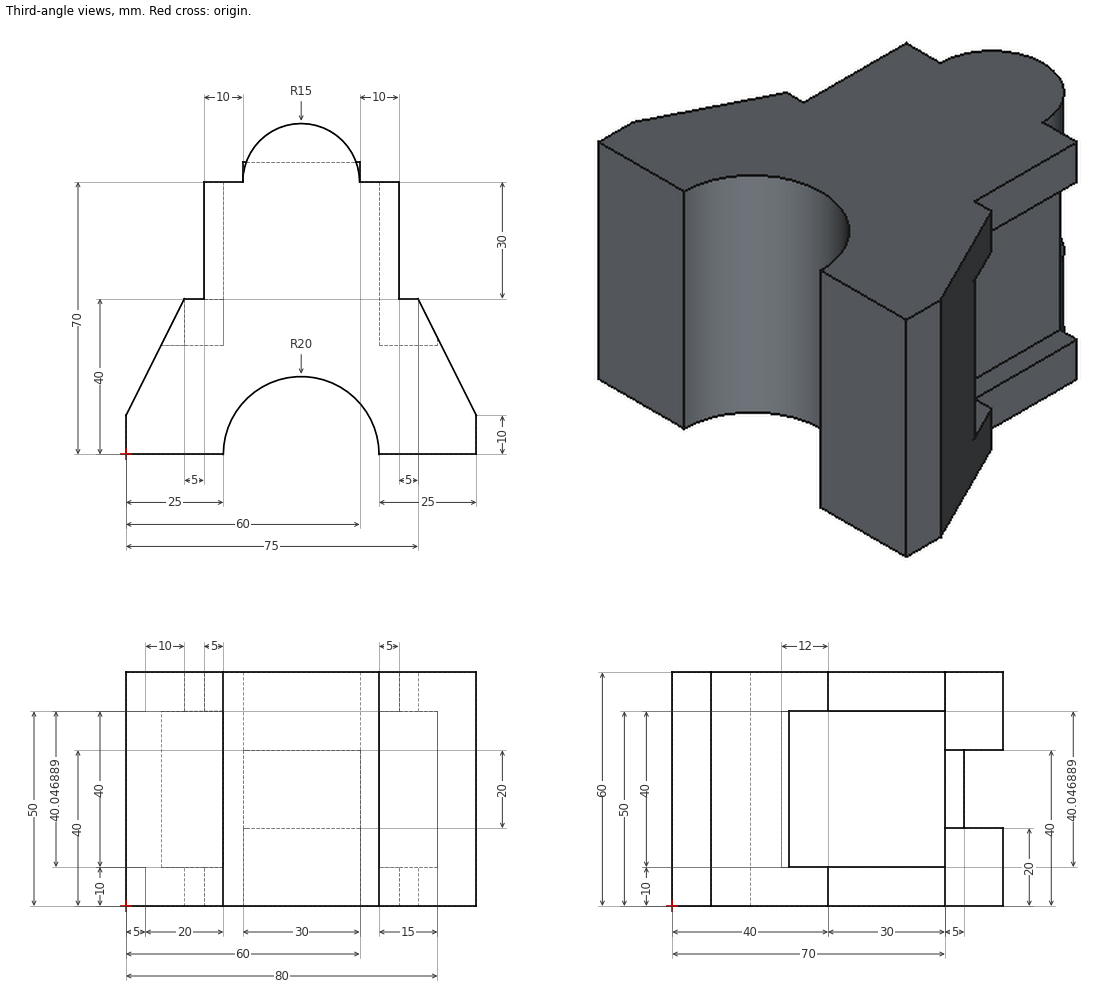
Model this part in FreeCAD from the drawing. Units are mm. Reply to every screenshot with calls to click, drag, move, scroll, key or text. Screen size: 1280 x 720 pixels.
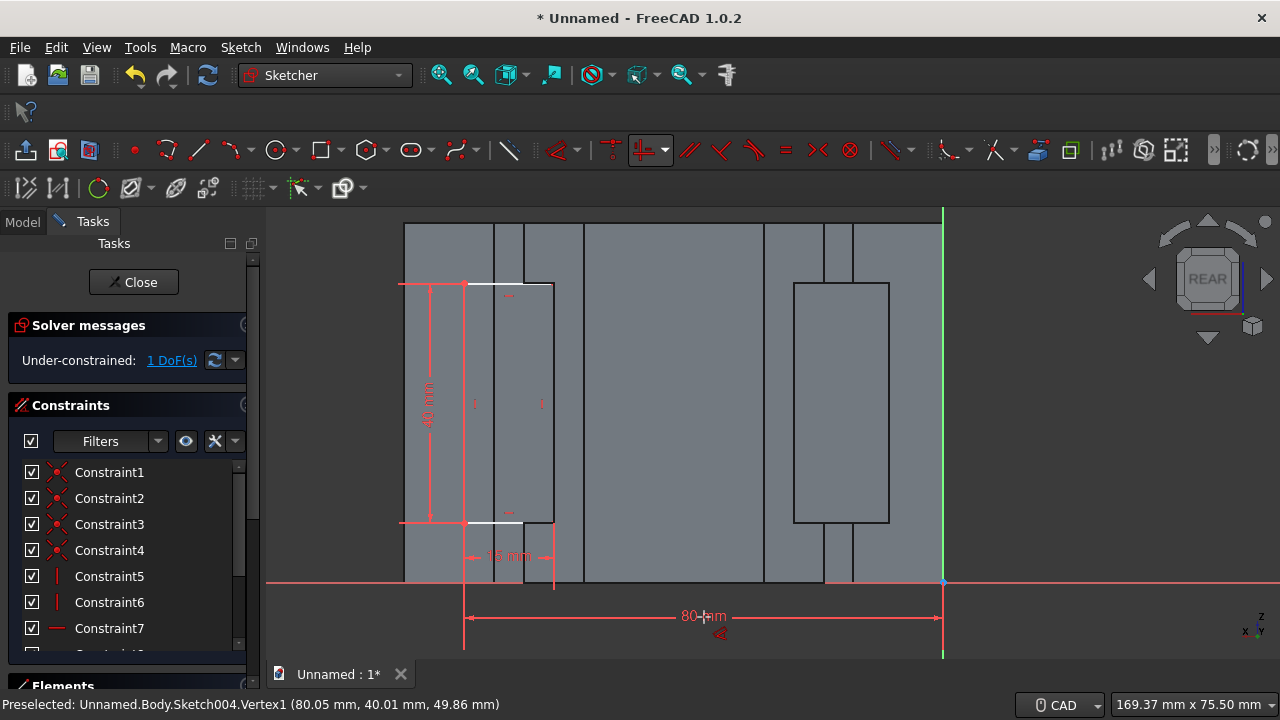
click(464, 284)
click(977, 433)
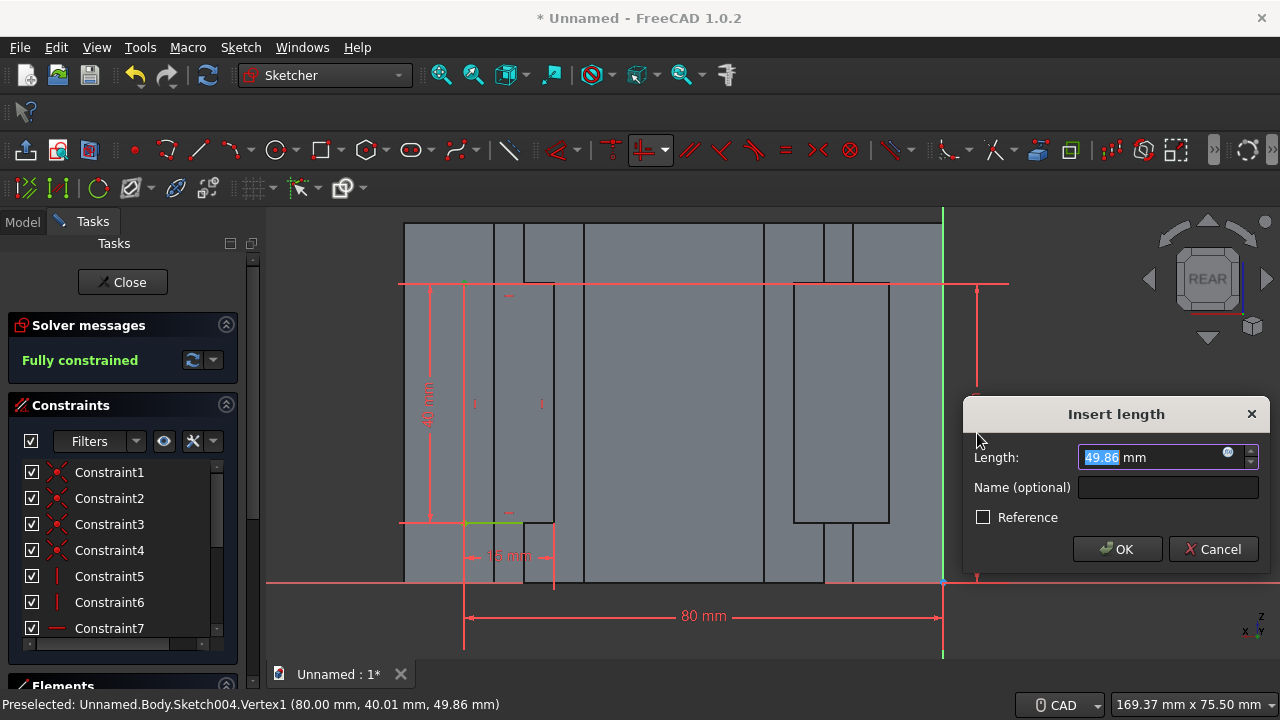
text(50)
key(Return)
key(Escape)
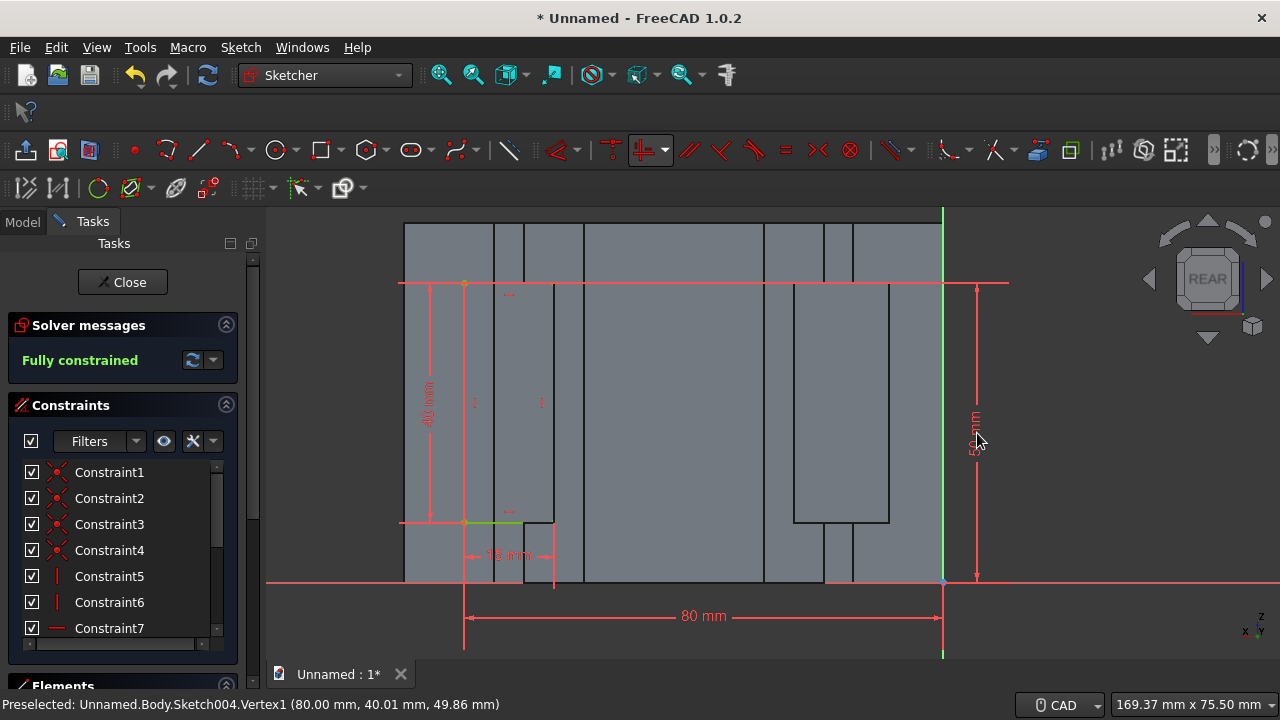
click(123, 282)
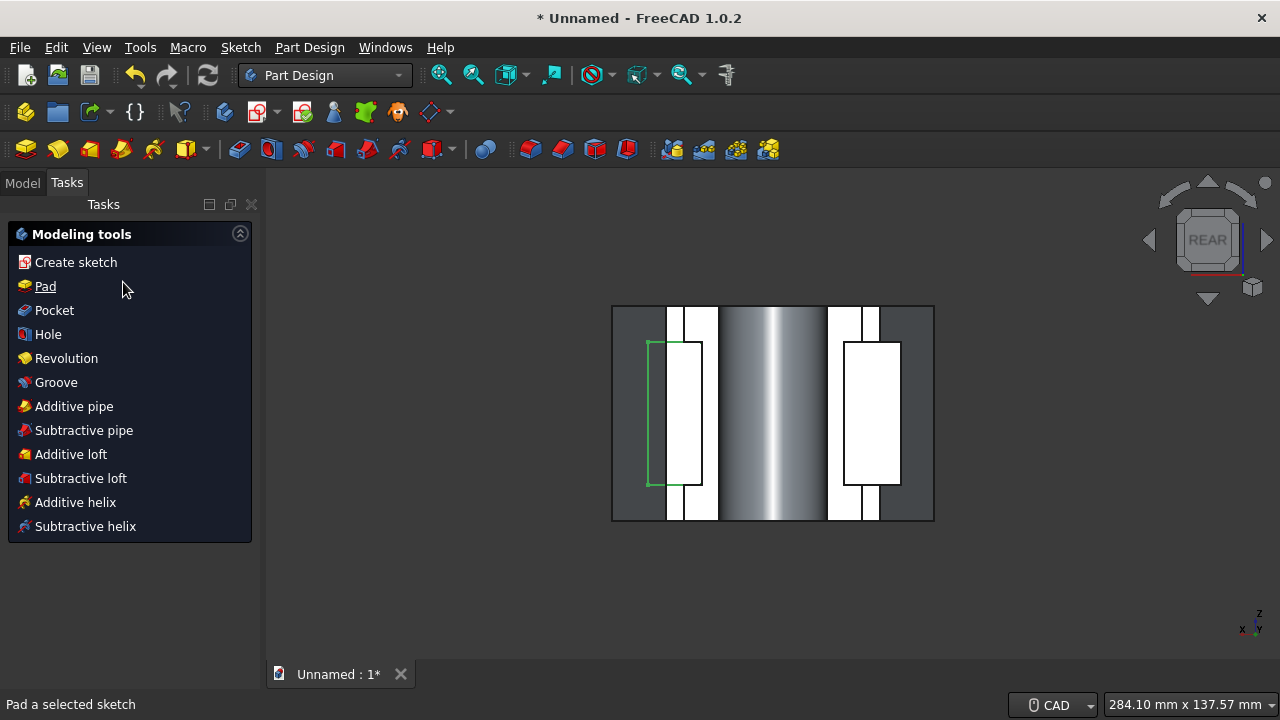
click(240, 150)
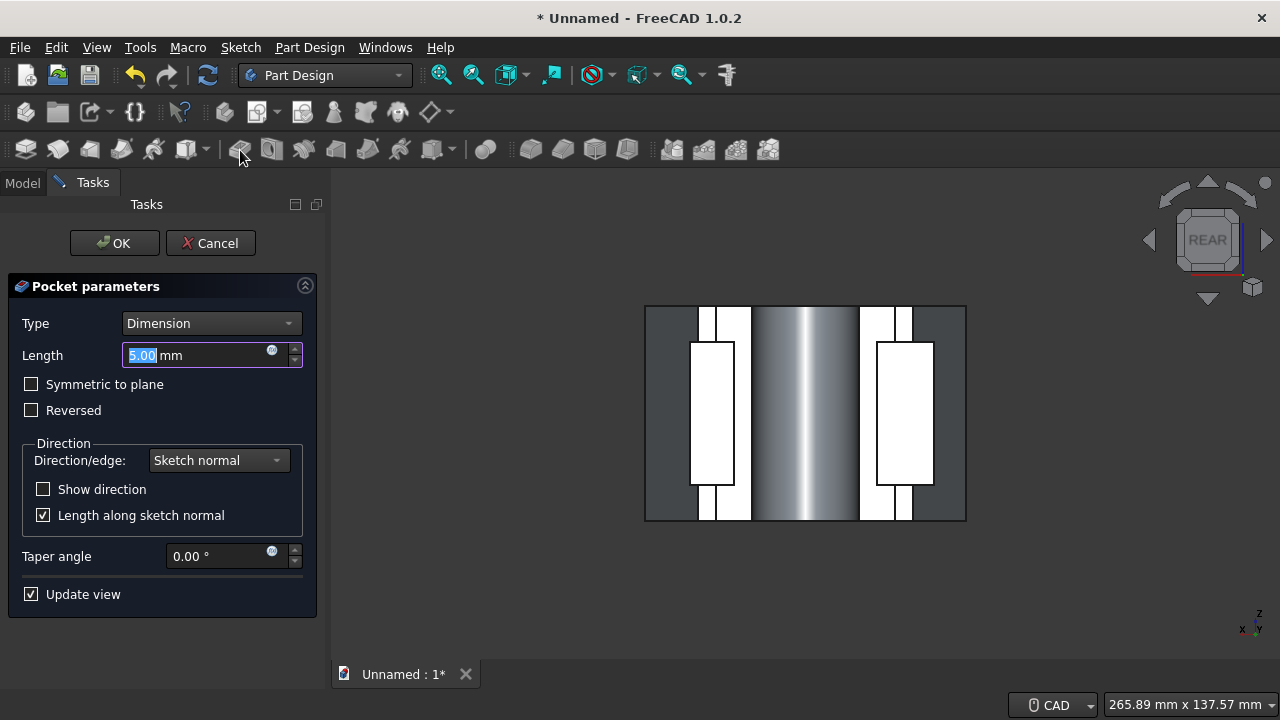
text(12)
key(Tab)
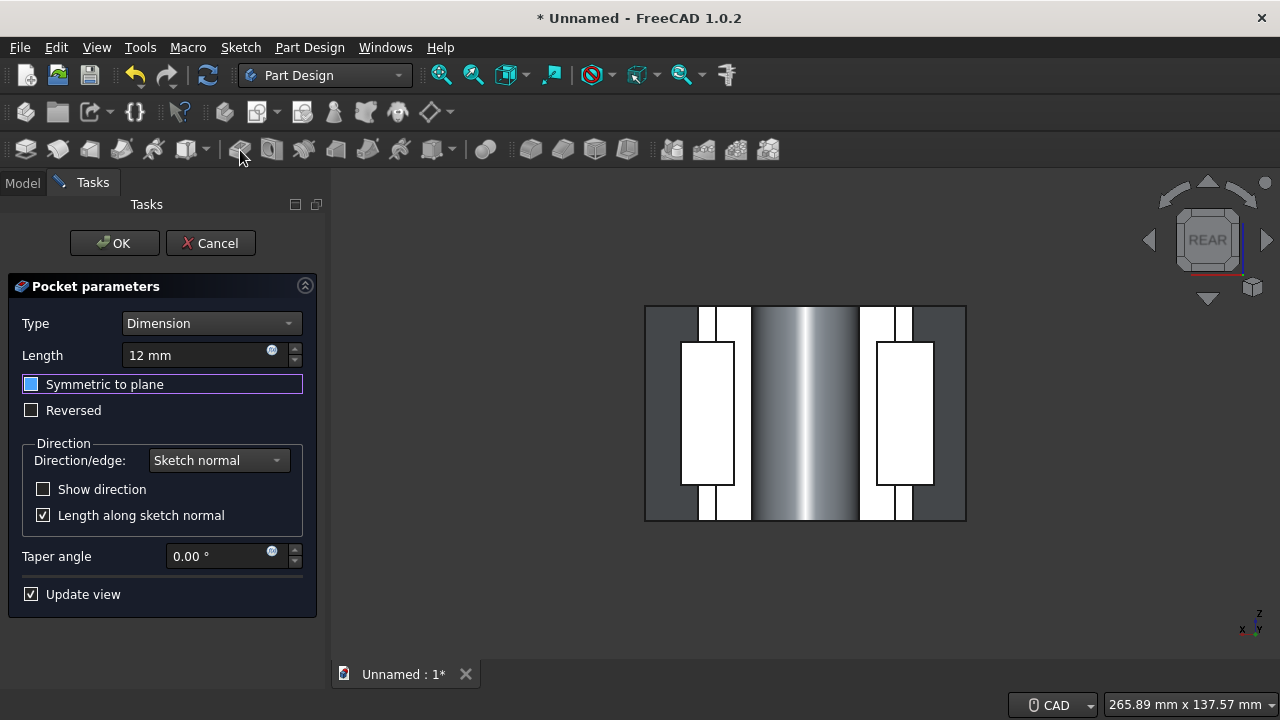
click(115, 243)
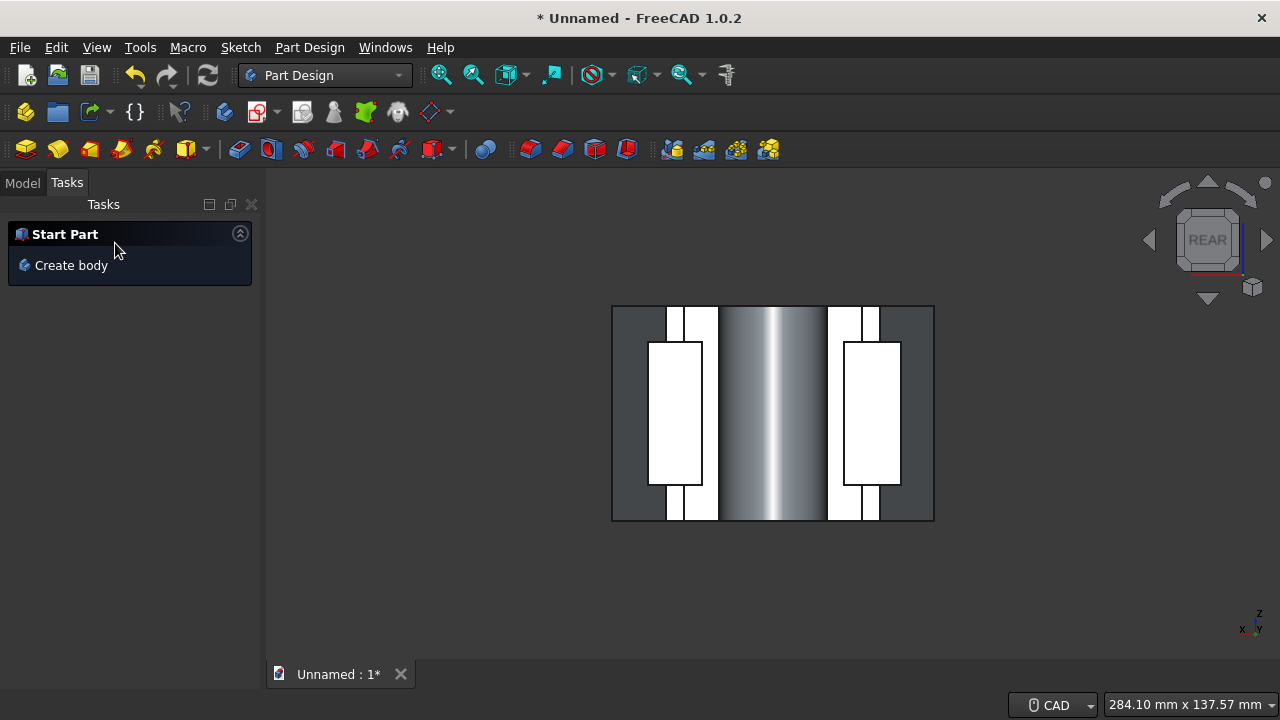
key(v)
key(f)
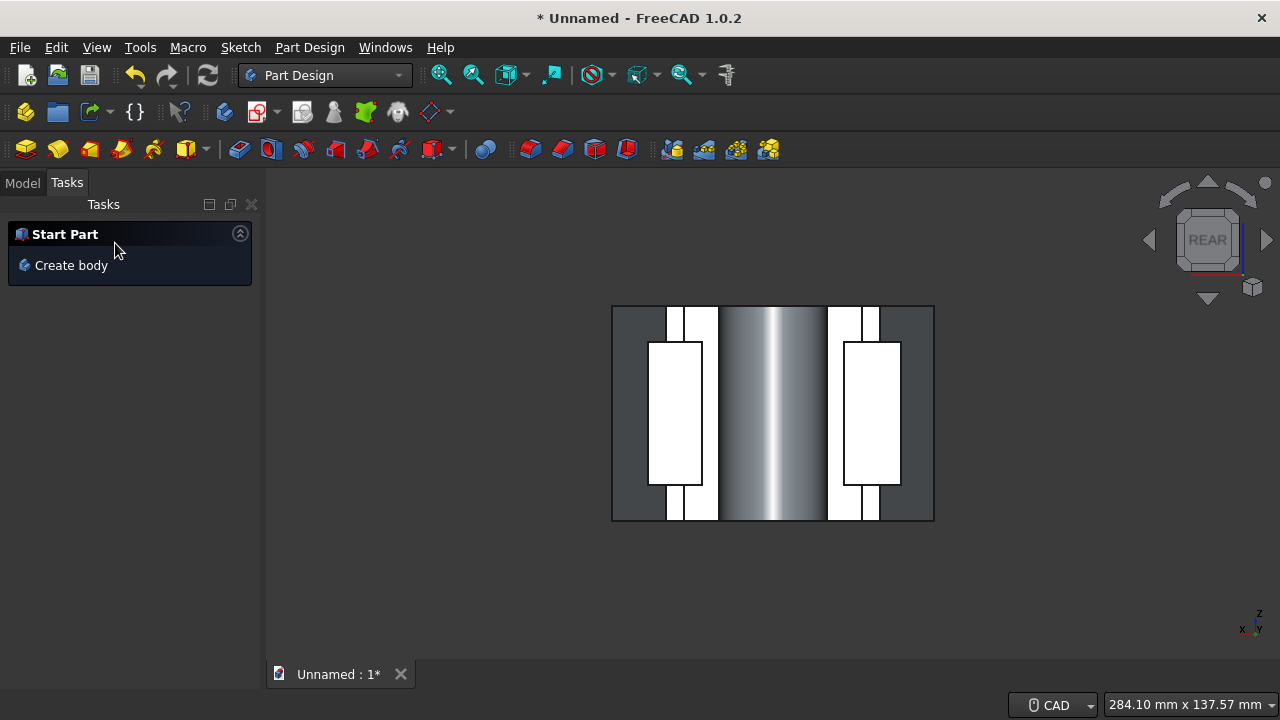
key(5)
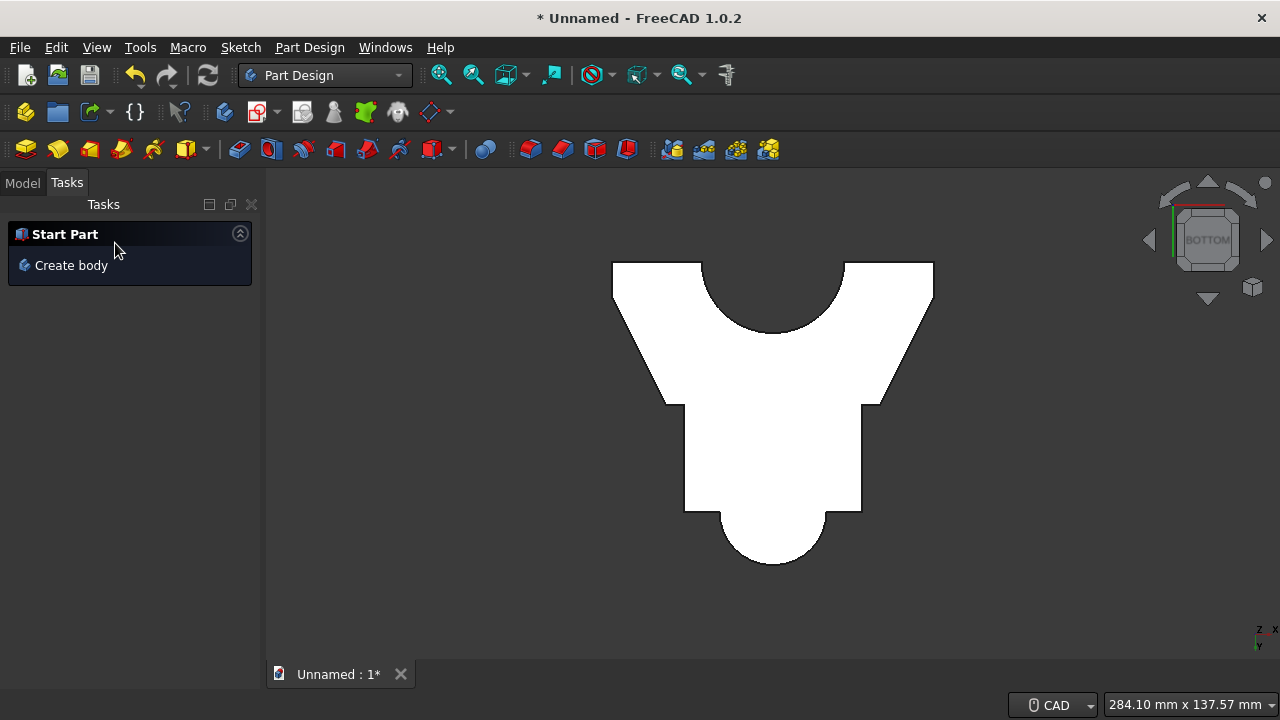
click(773, 412)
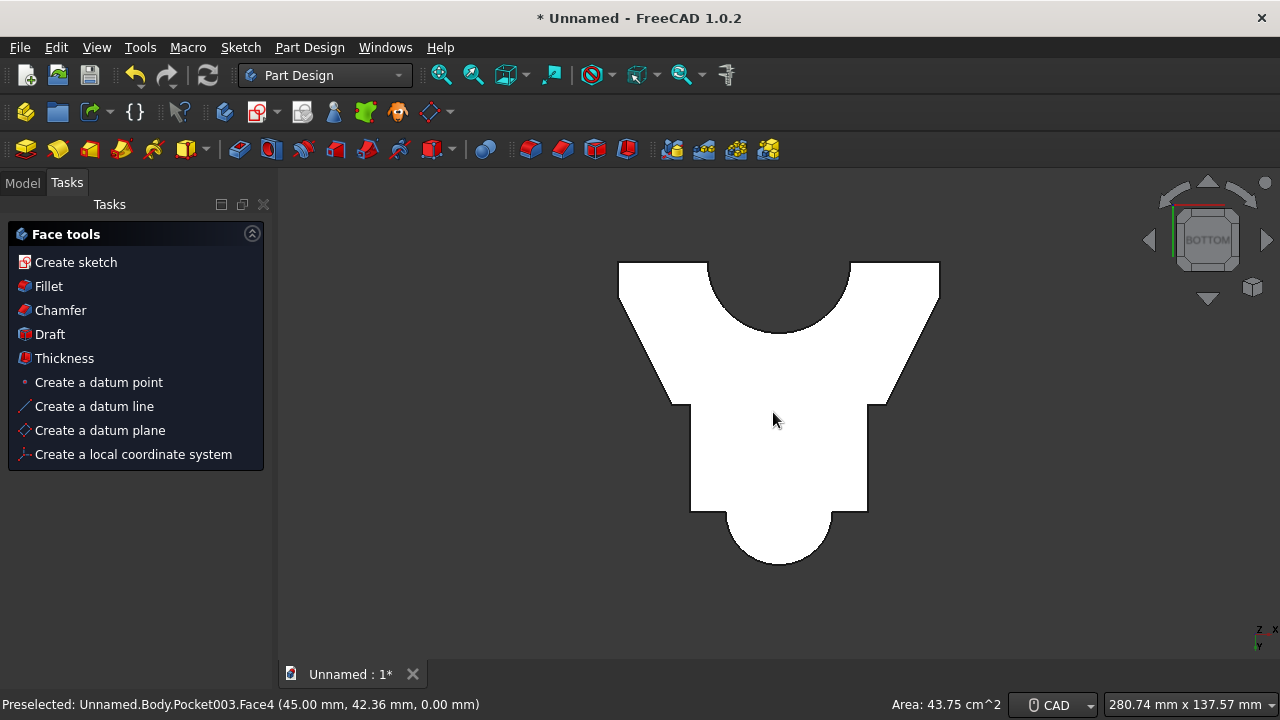
click(258, 112)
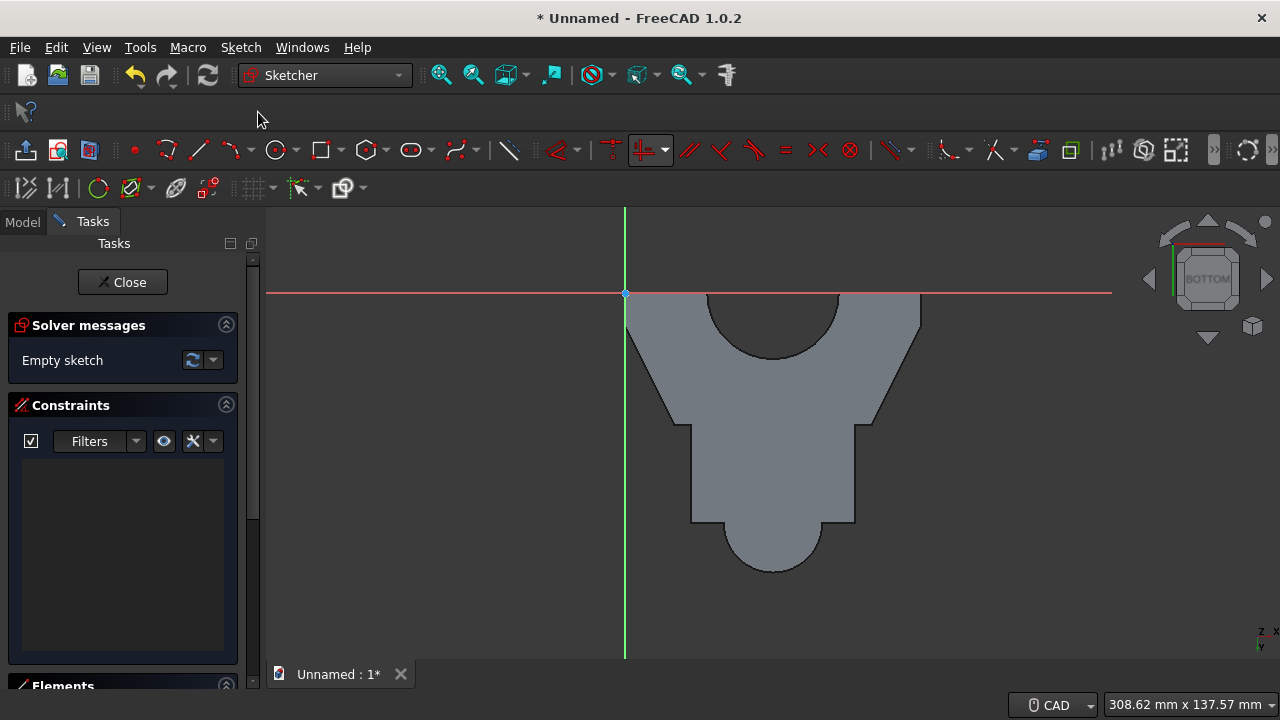
scroll(787, 571, up, 9)